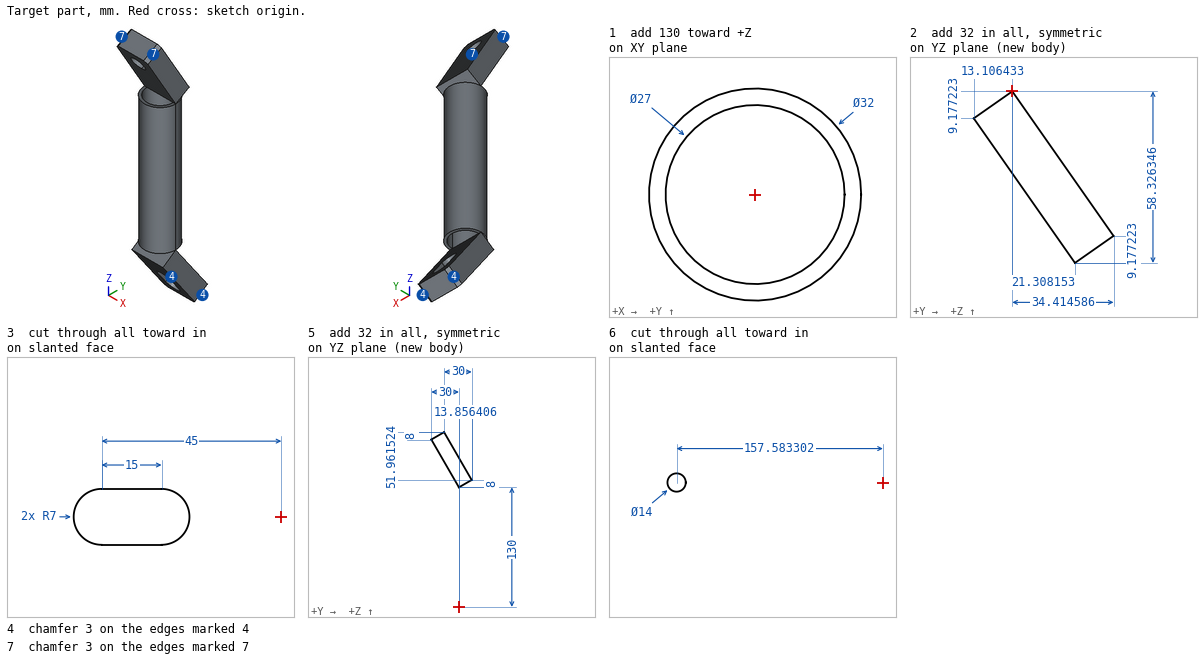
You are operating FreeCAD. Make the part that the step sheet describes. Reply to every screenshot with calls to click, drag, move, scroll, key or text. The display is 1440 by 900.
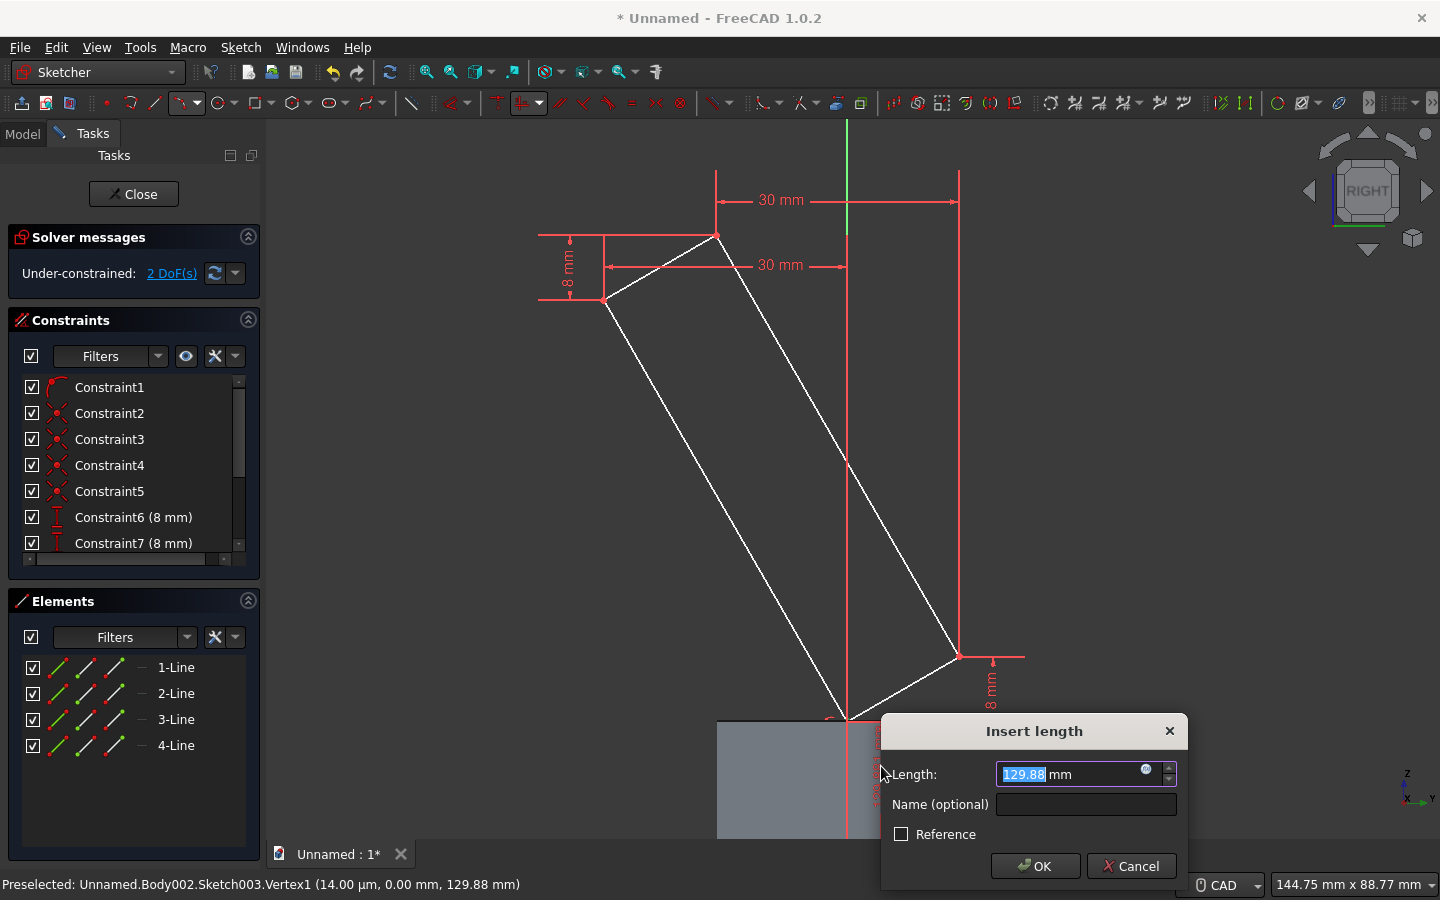
text(130)
key(Return)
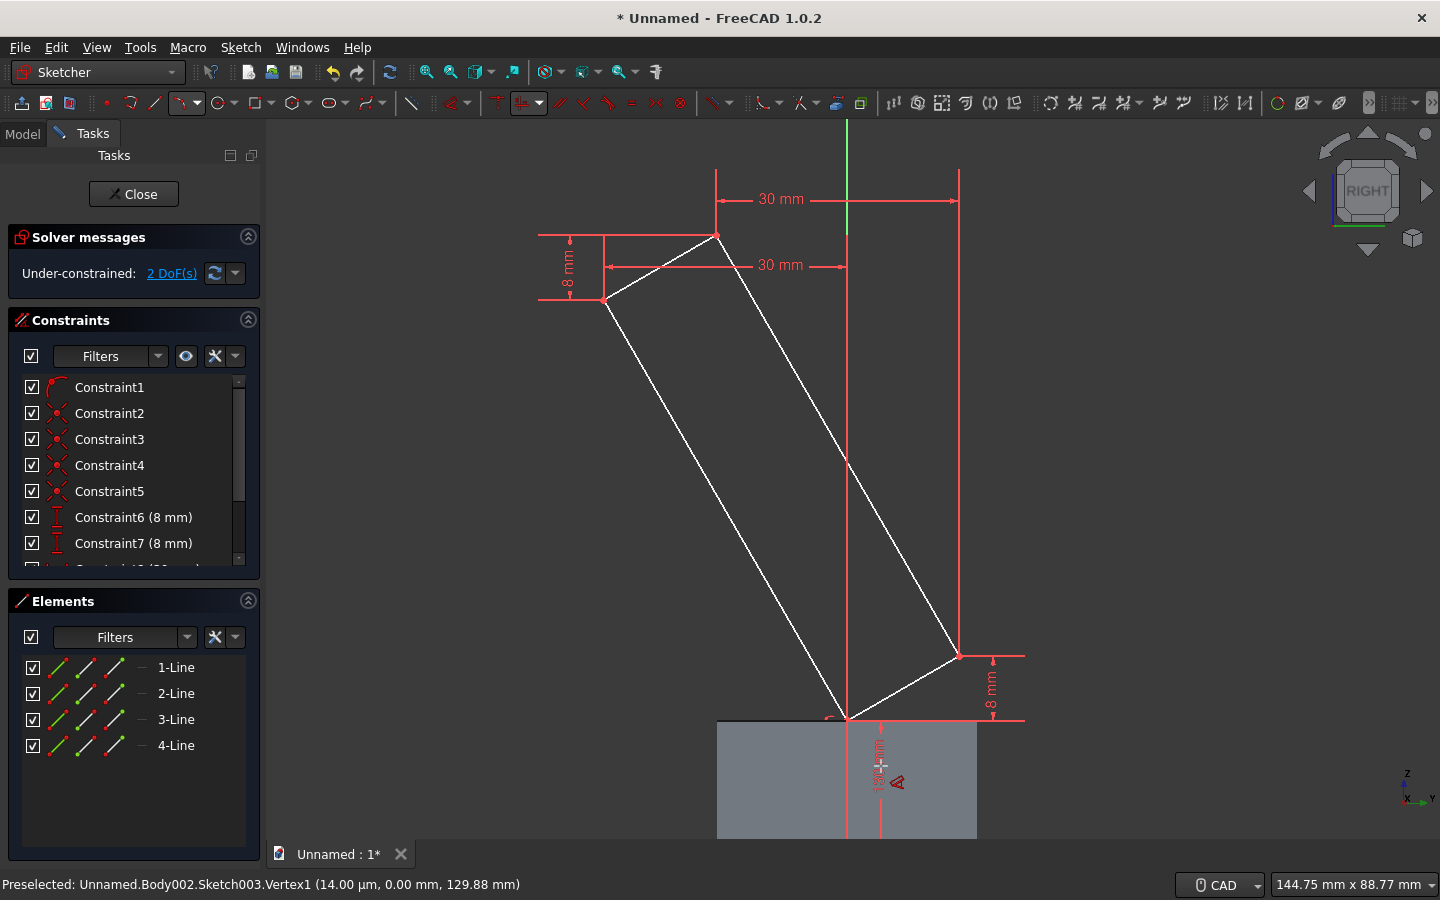
click(959, 656)
click(903, 622)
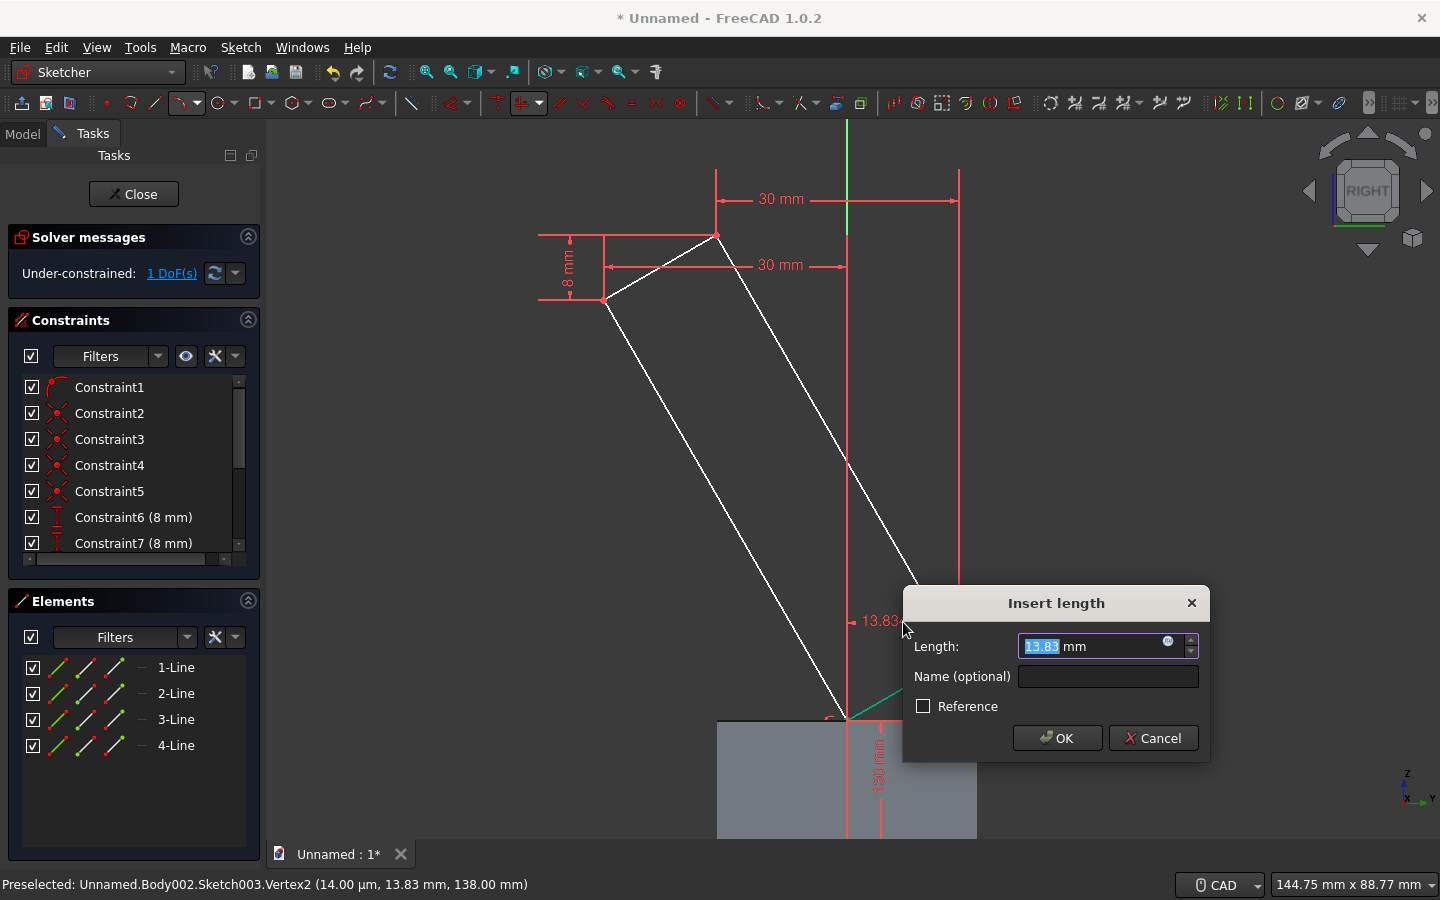
text(13.856406)
key(Return)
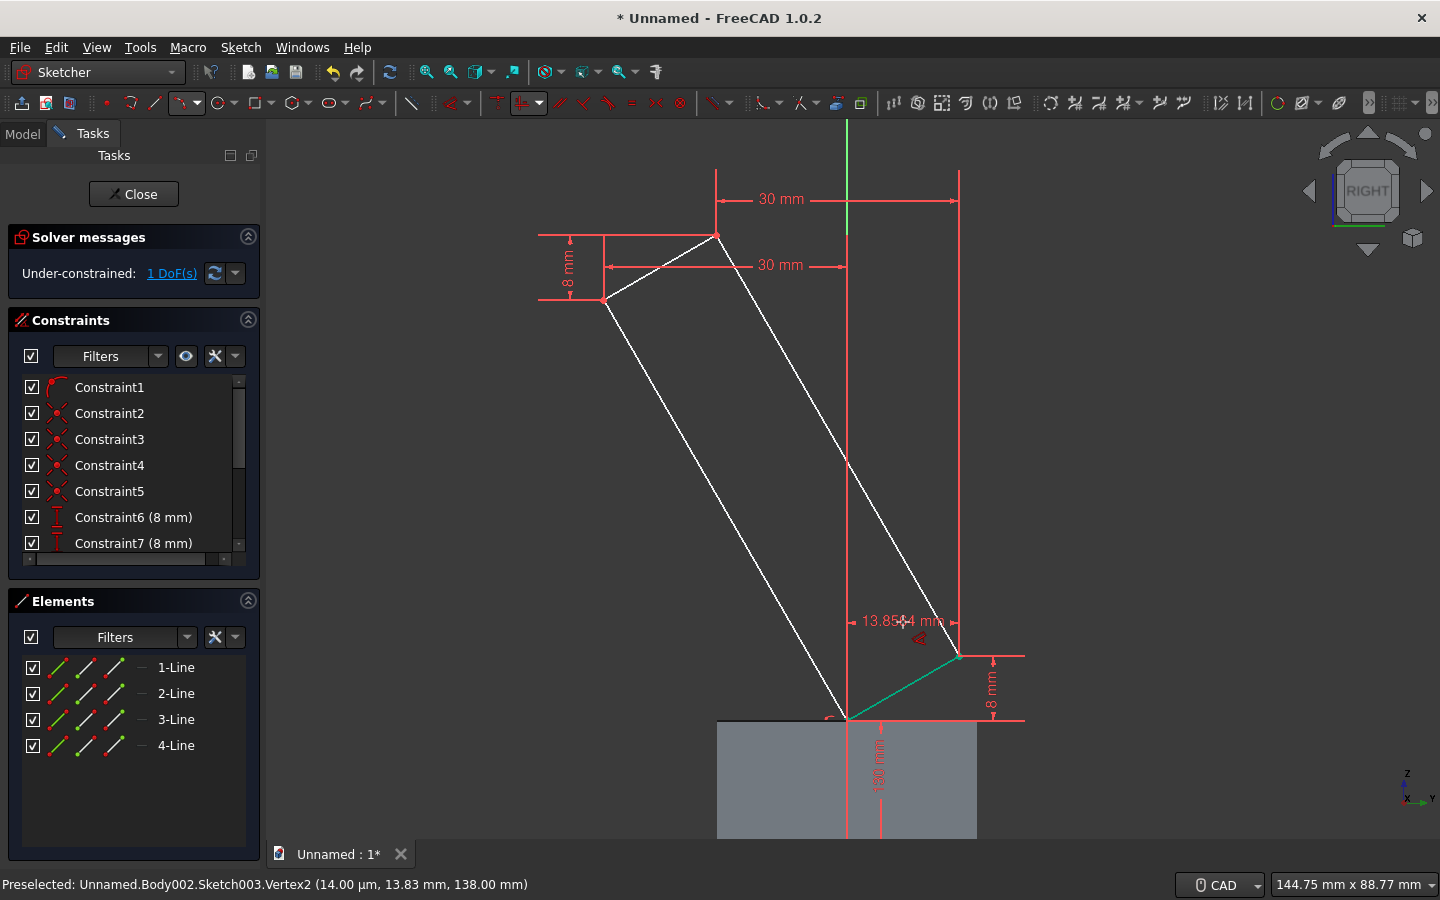
click(887, 530)
click(994, 446)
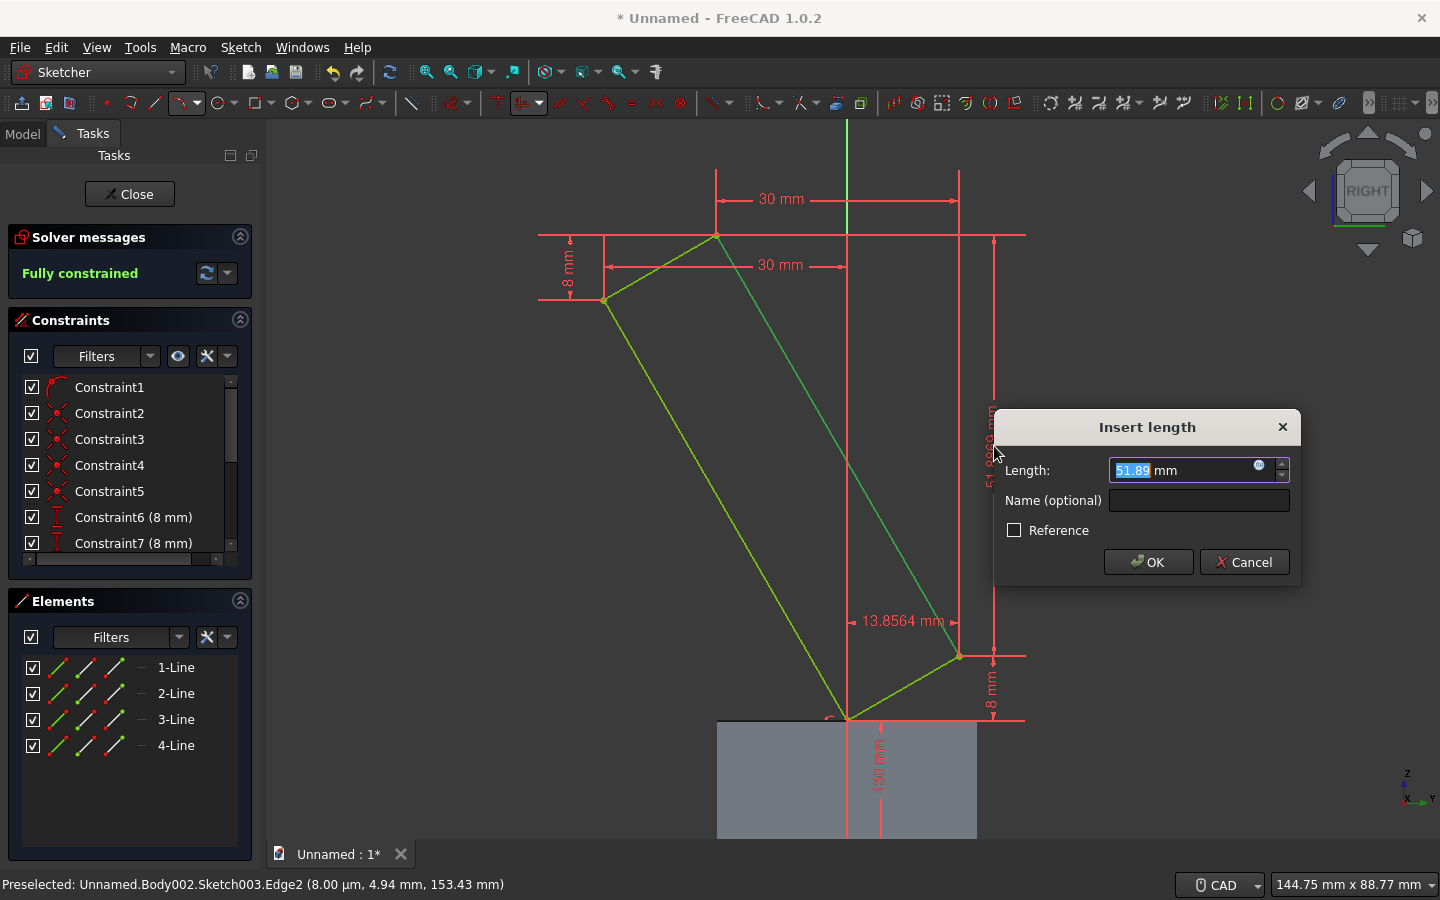
text(51.961524)
key(Return)
key(Escape)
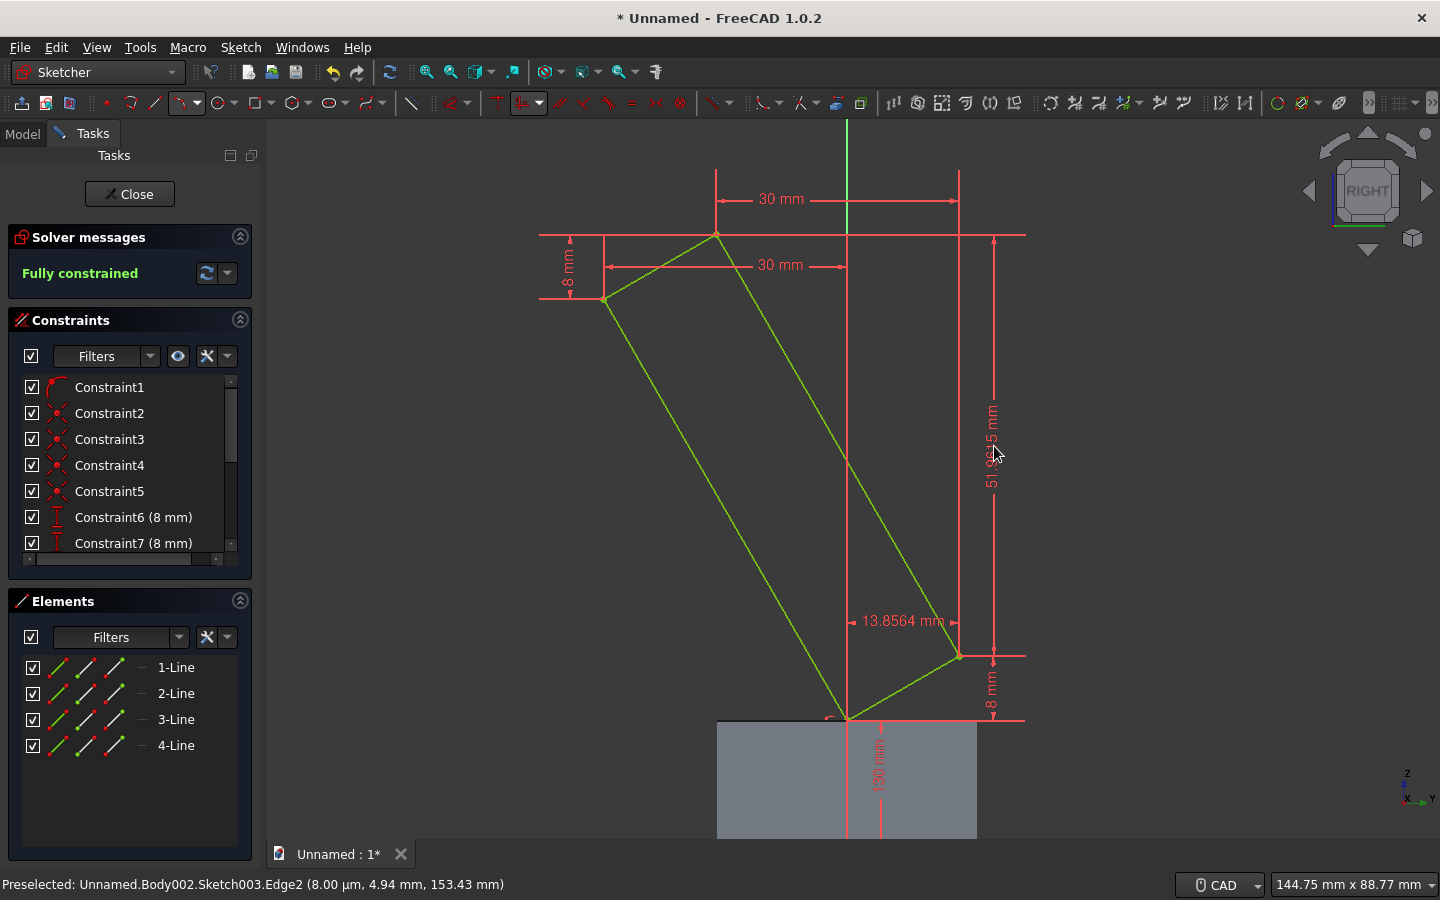
click(130, 194)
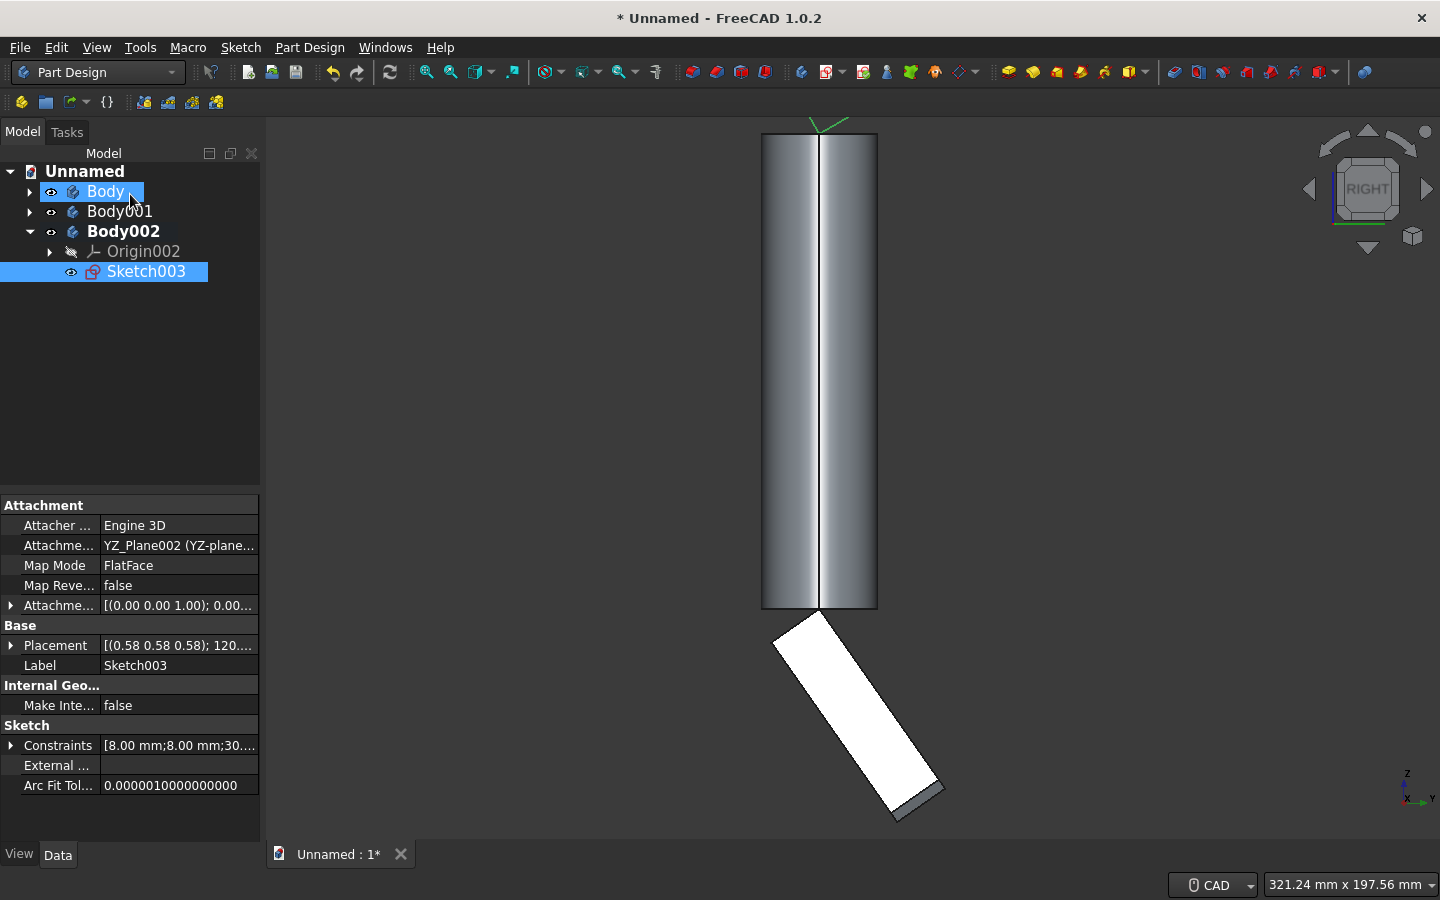
click(1010, 72)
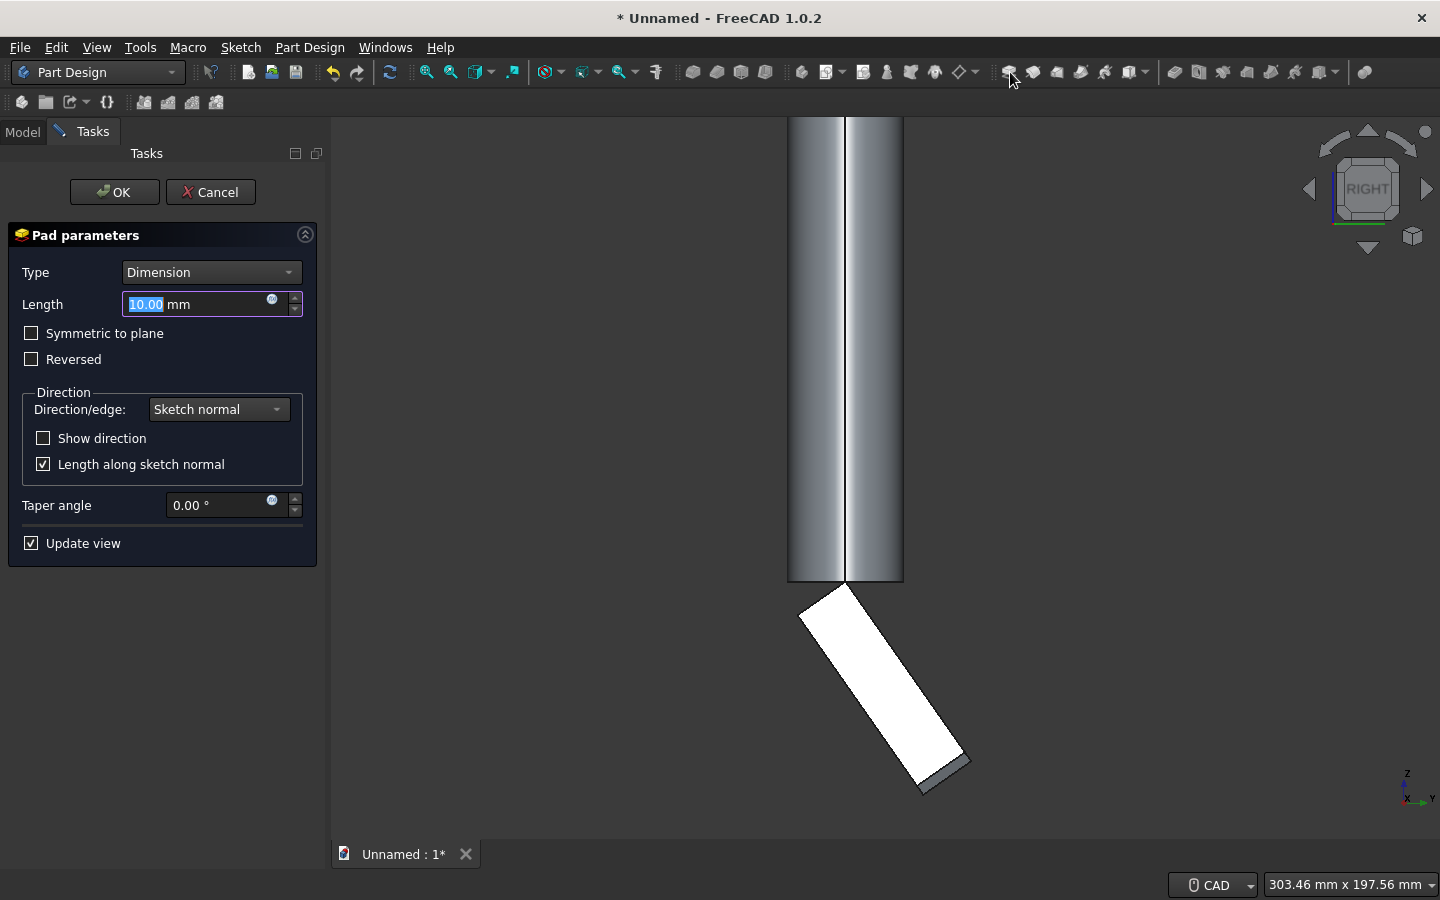
text(32)
key(Tab)